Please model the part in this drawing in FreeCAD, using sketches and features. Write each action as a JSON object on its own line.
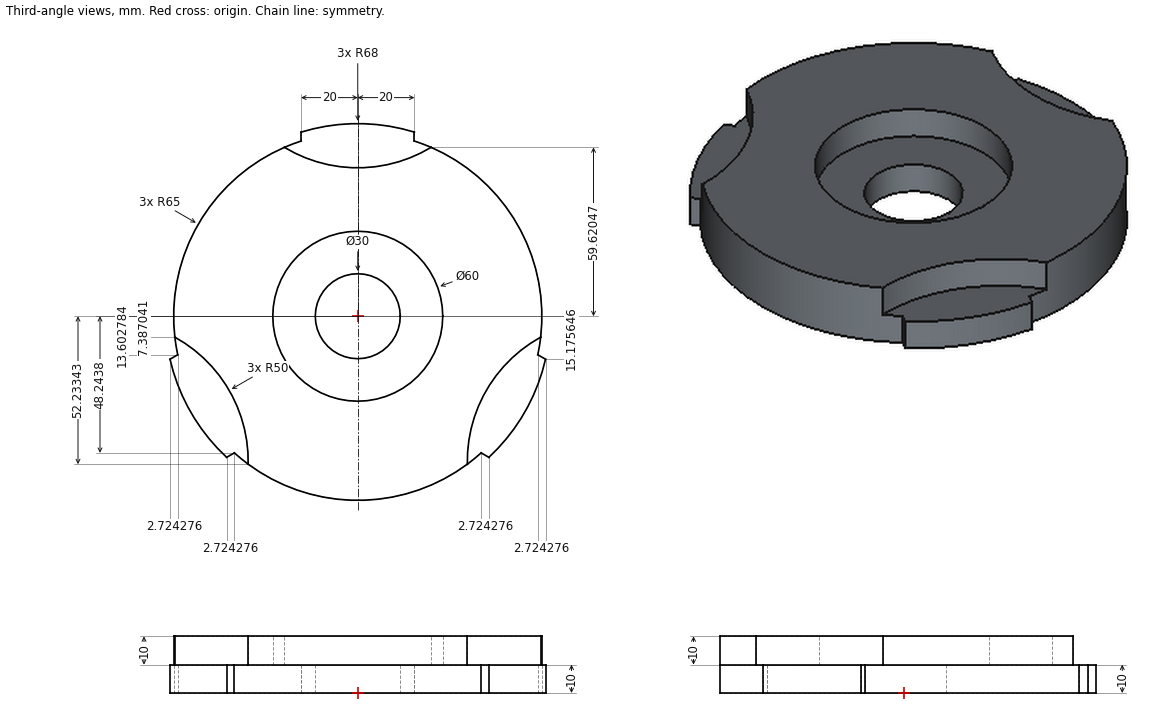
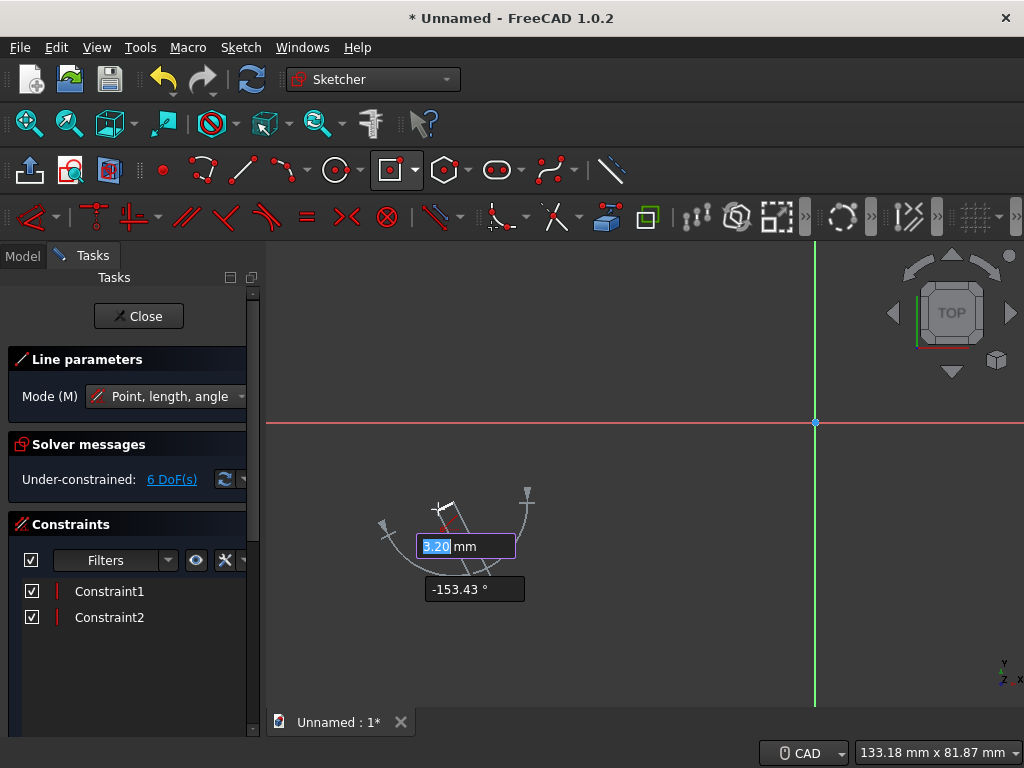
{"action": "left_click", "coordinate": [438, 509]}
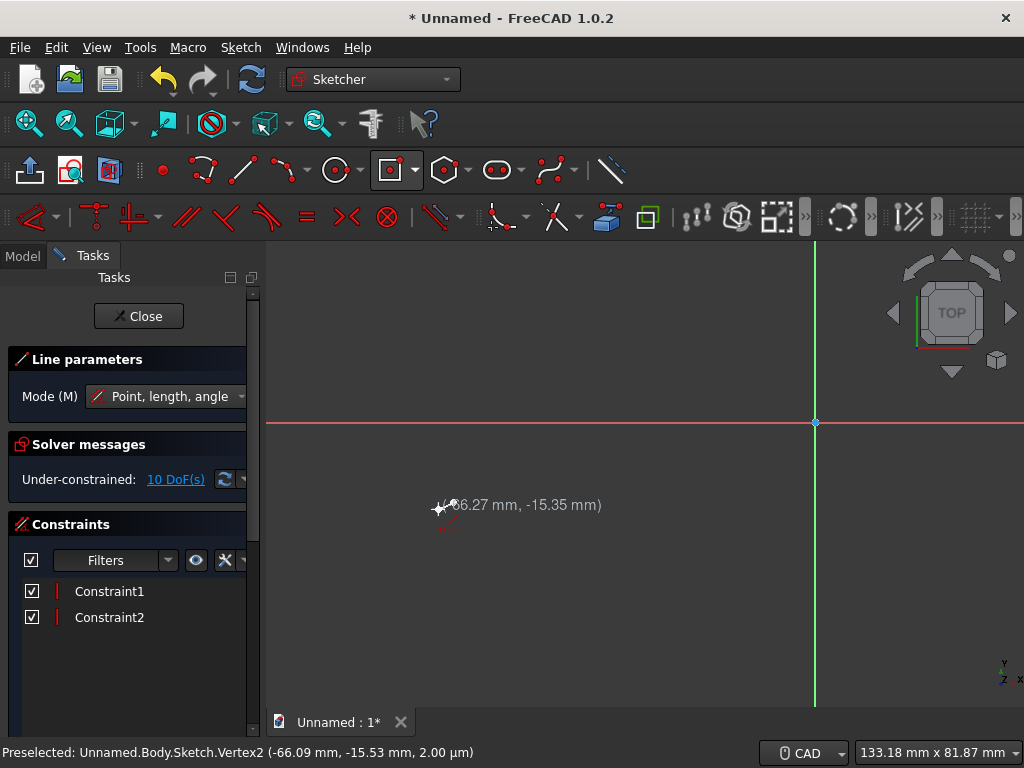
{"action": "scroll", "coordinate": [438, 509], "scroll_direction": "down", "scroll_amount": 5}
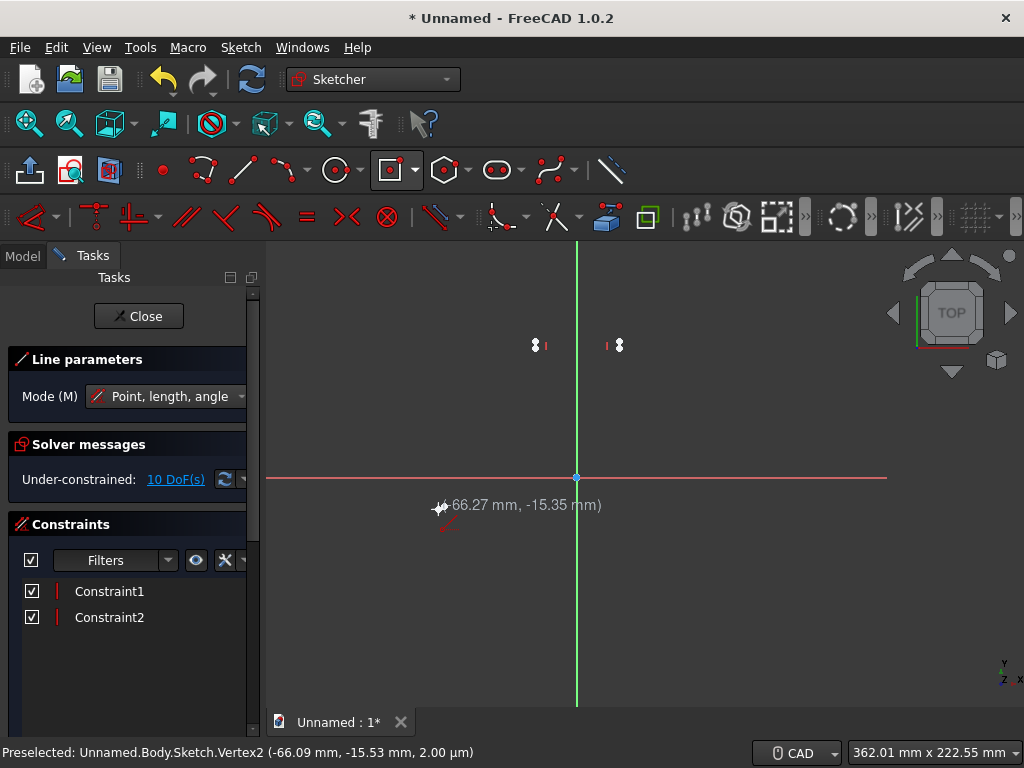
{"action": "left_click", "coordinate": [480, 582]}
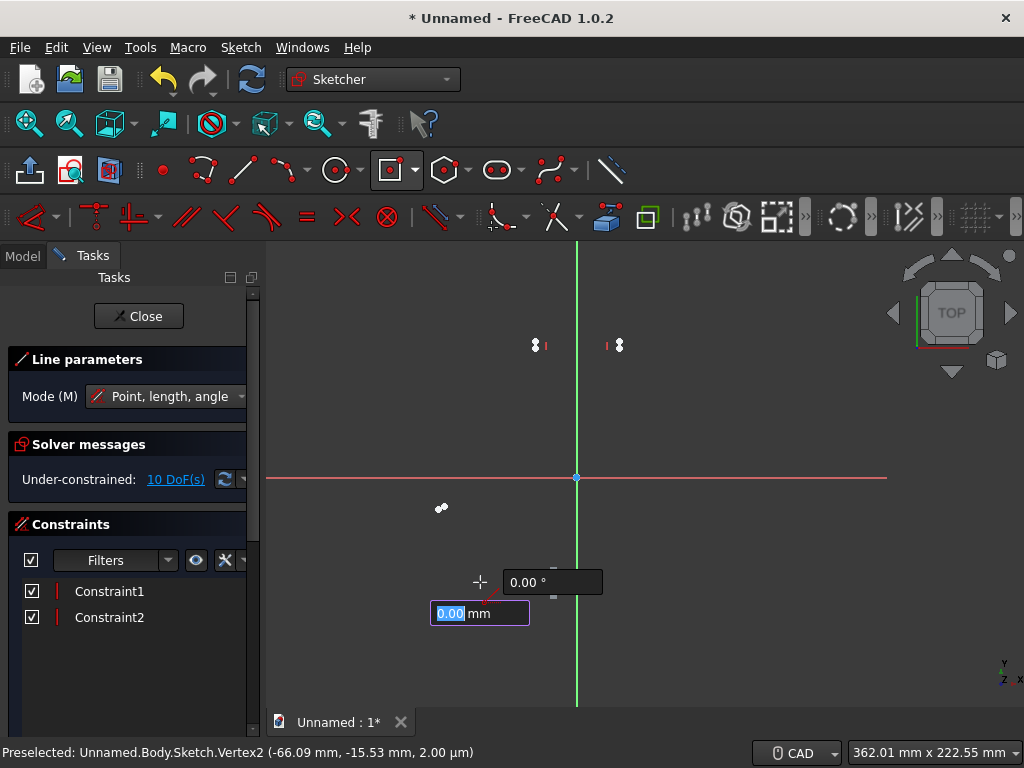
{"action": "scroll", "coordinate": [486, 579], "scroll_direction": "up", "scroll_amount": 5}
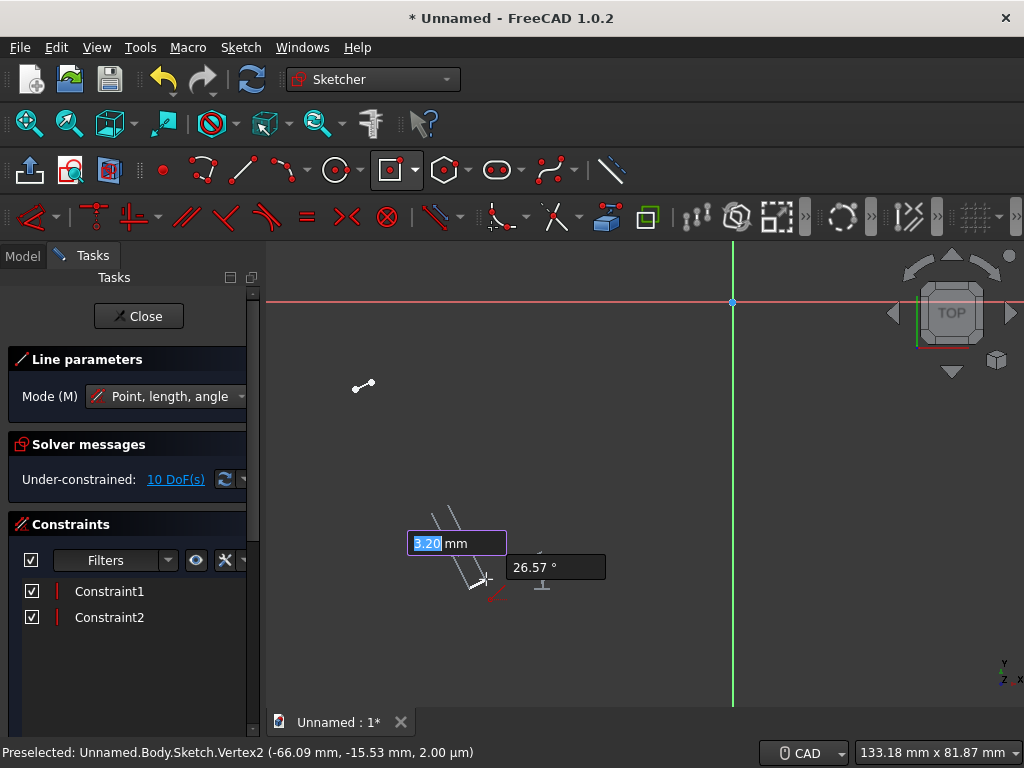
{"action": "left_click", "coordinate": [485, 577]}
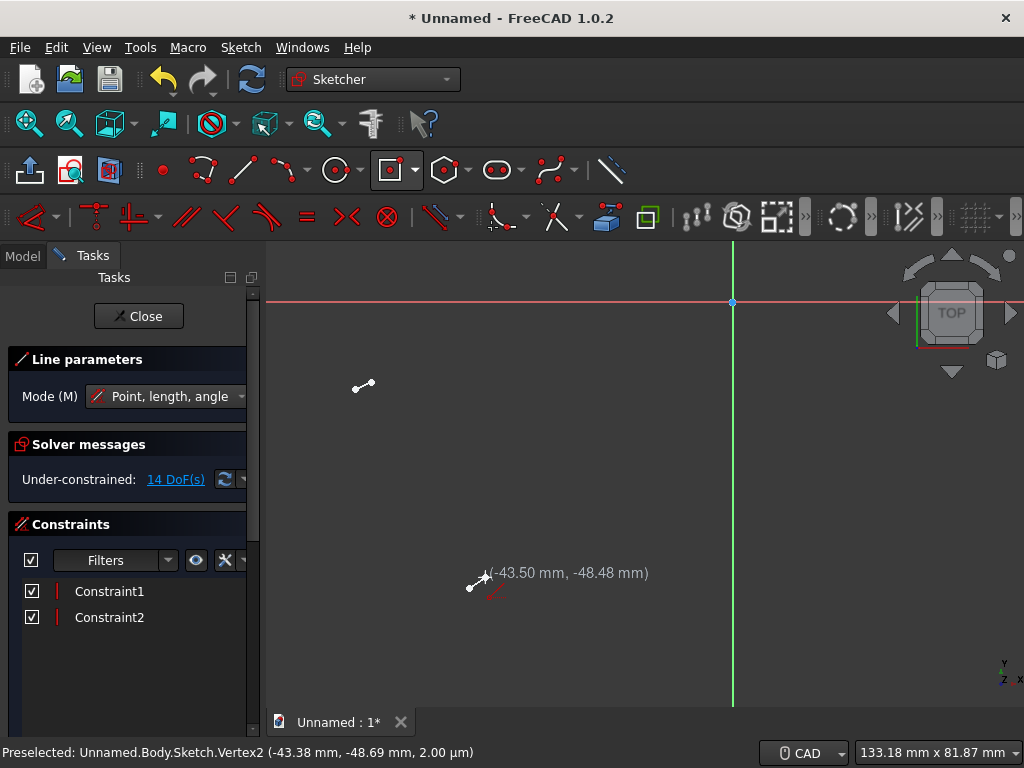
{"action": "scroll", "coordinate": [486, 579], "scroll_direction": "down", "scroll_amount": 5}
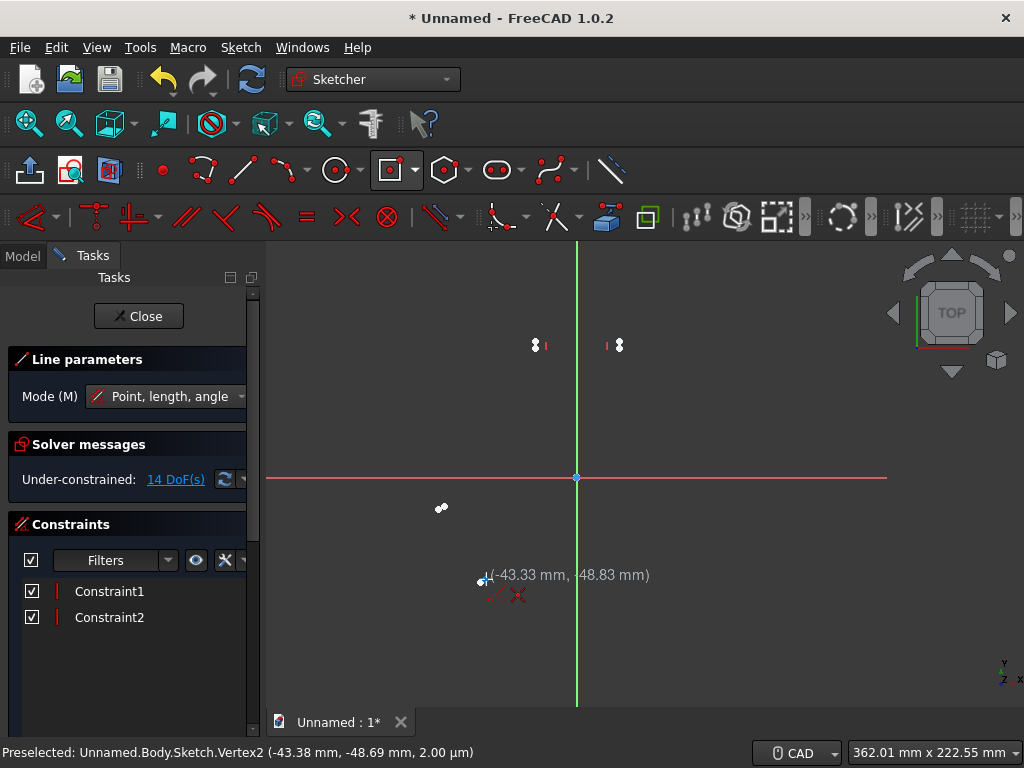
{"action": "left_click", "coordinate": [668, 579]}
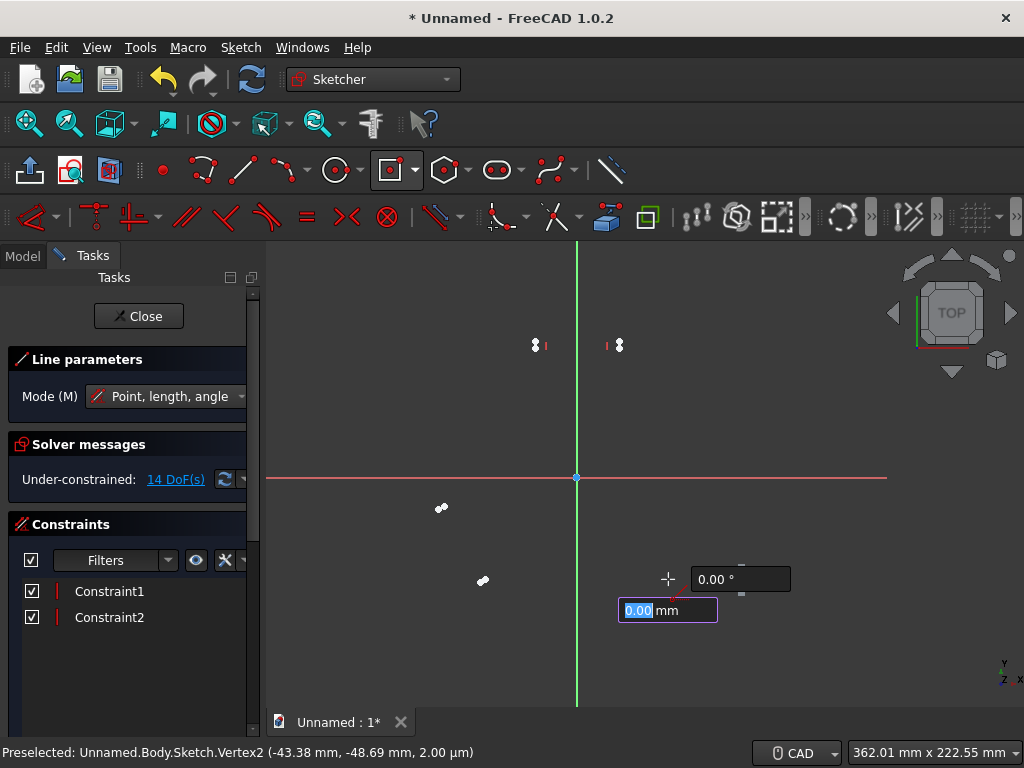
{"action": "scroll", "coordinate": [674, 582], "scroll_direction": "up", "scroll_amount": 5}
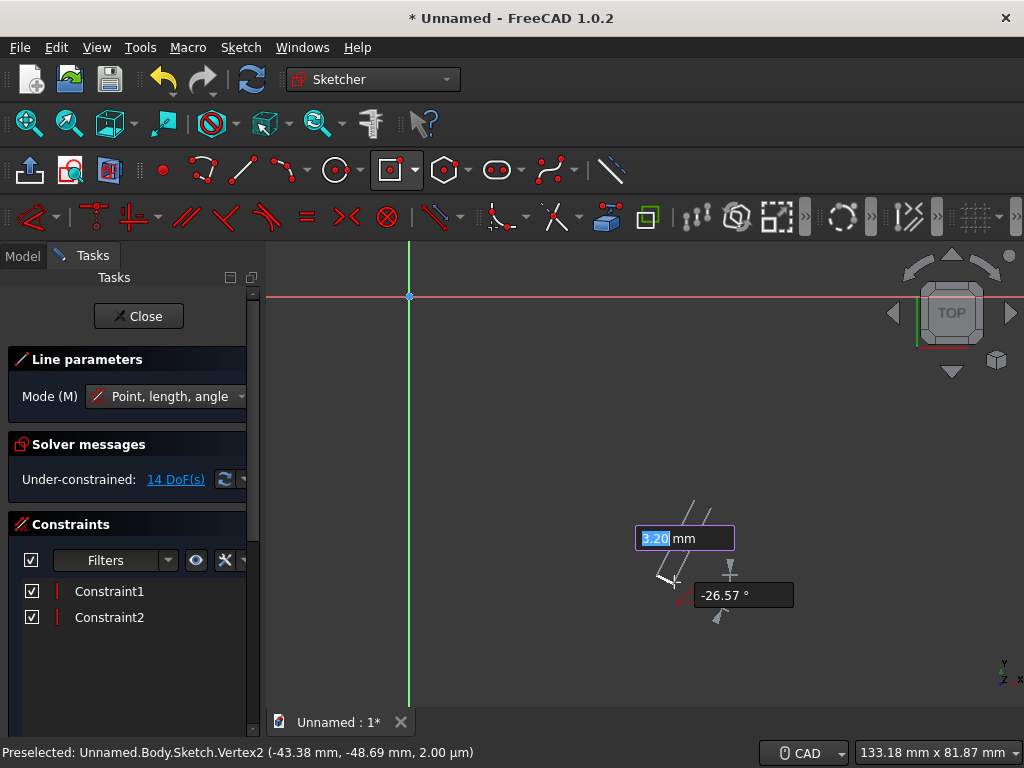
{"action": "left_click", "coordinate": [673, 580]}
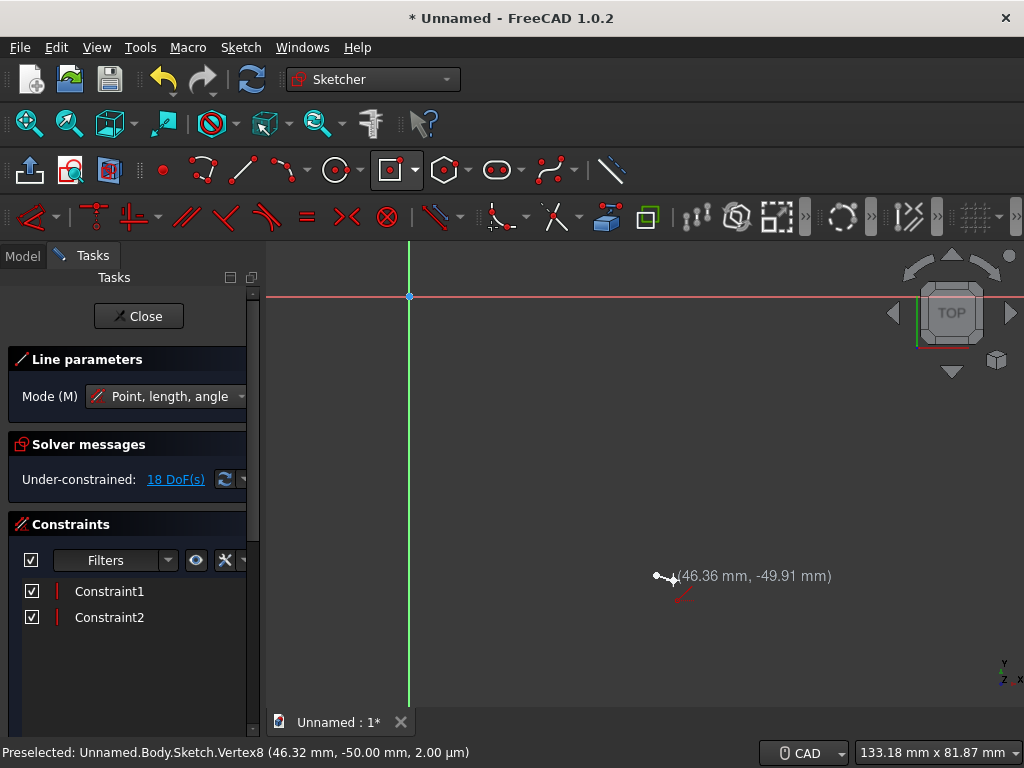
{"action": "left_click", "coordinate": [786, 383]}
{"action": "left_click", "coordinate": [771, 374]}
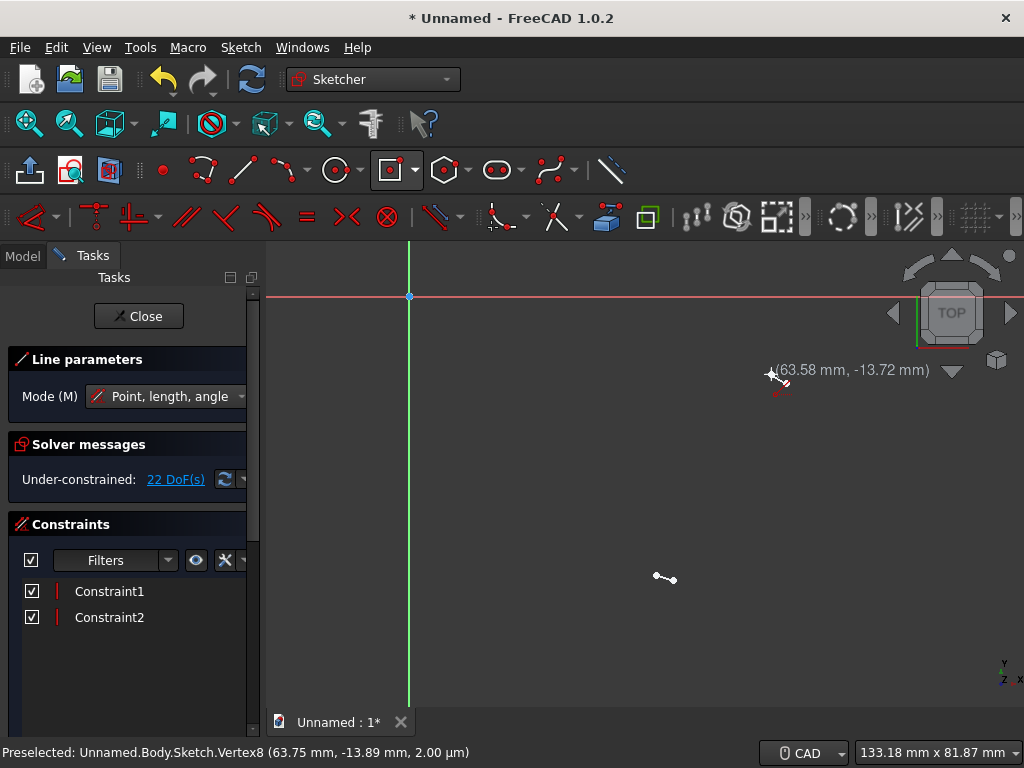
{"action": "left_click", "coordinate": [284, 170]}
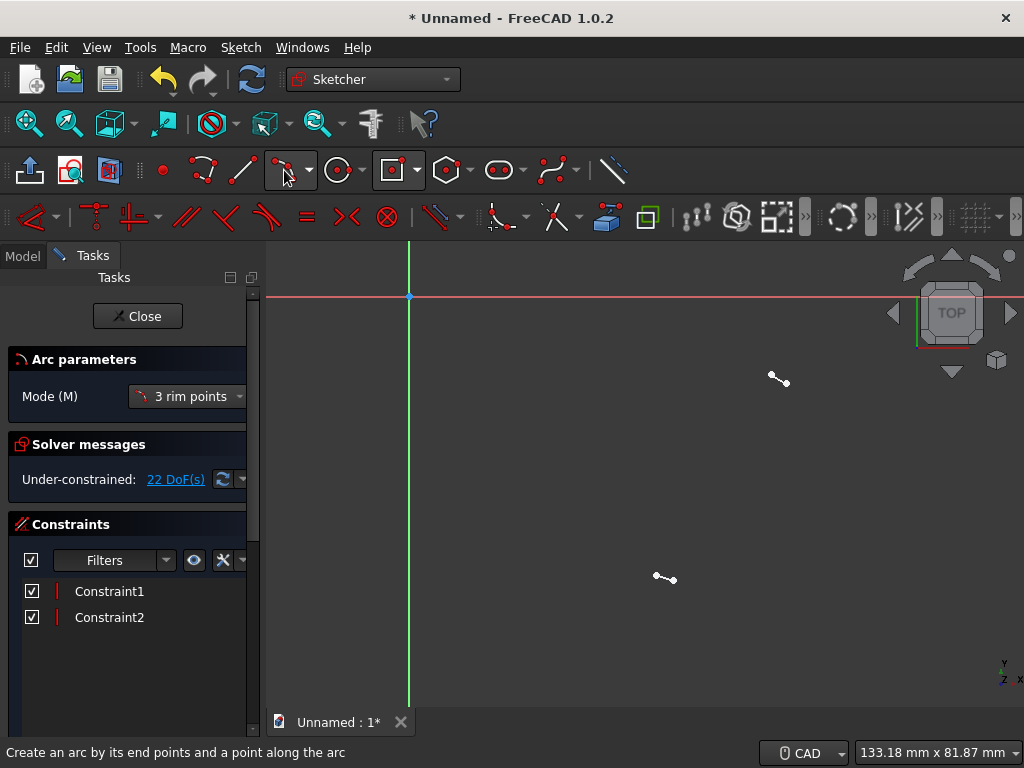
{"action": "scroll", "coordinate": [674, 582], "scroll_direction": "down", "scroll_amount": 5}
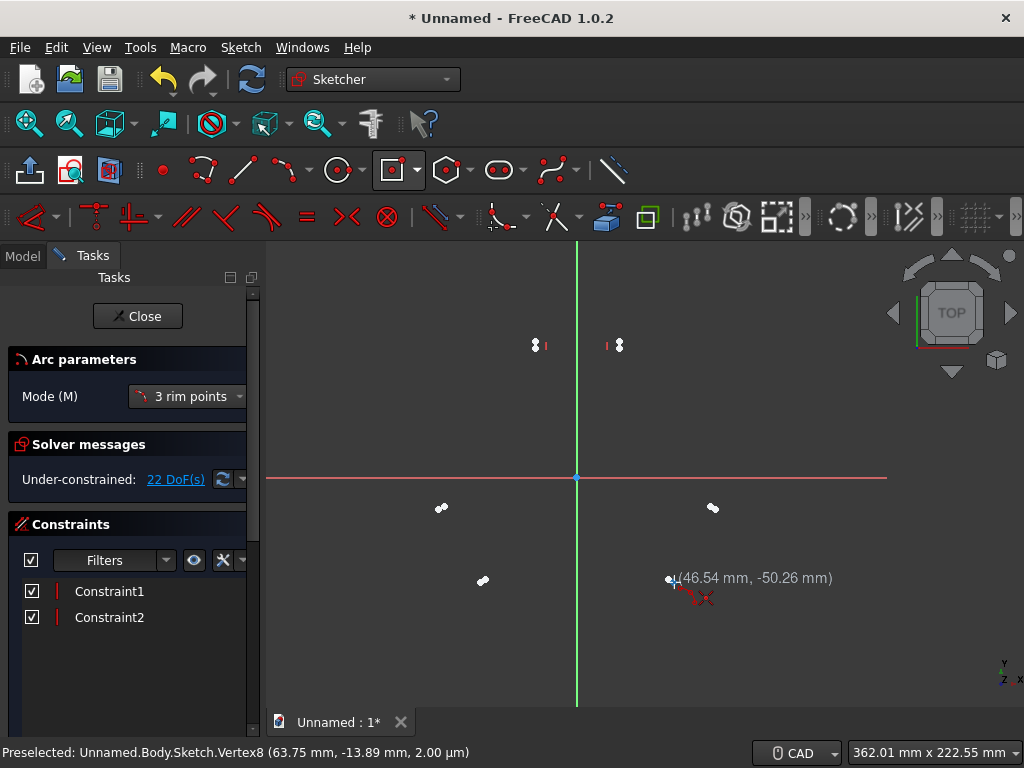
{"action": "scroll", "coordinate": [619, 342], "scroll_direction": "up", "scroll_amount": 8}